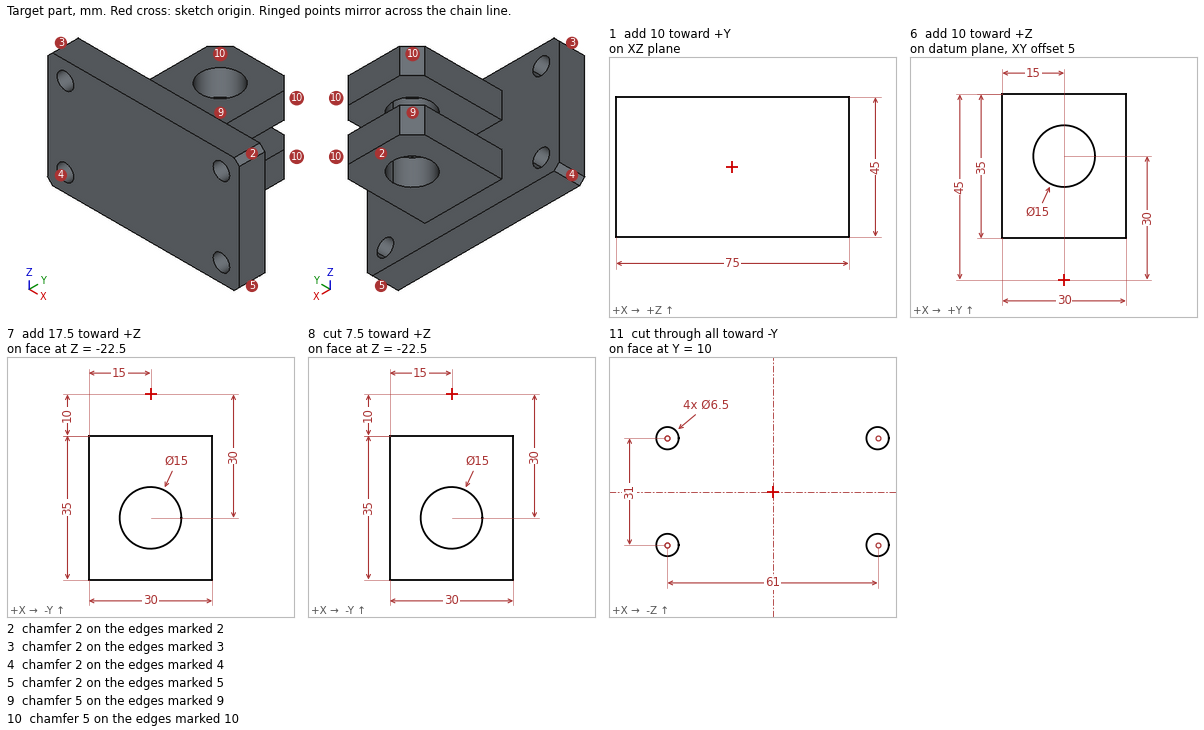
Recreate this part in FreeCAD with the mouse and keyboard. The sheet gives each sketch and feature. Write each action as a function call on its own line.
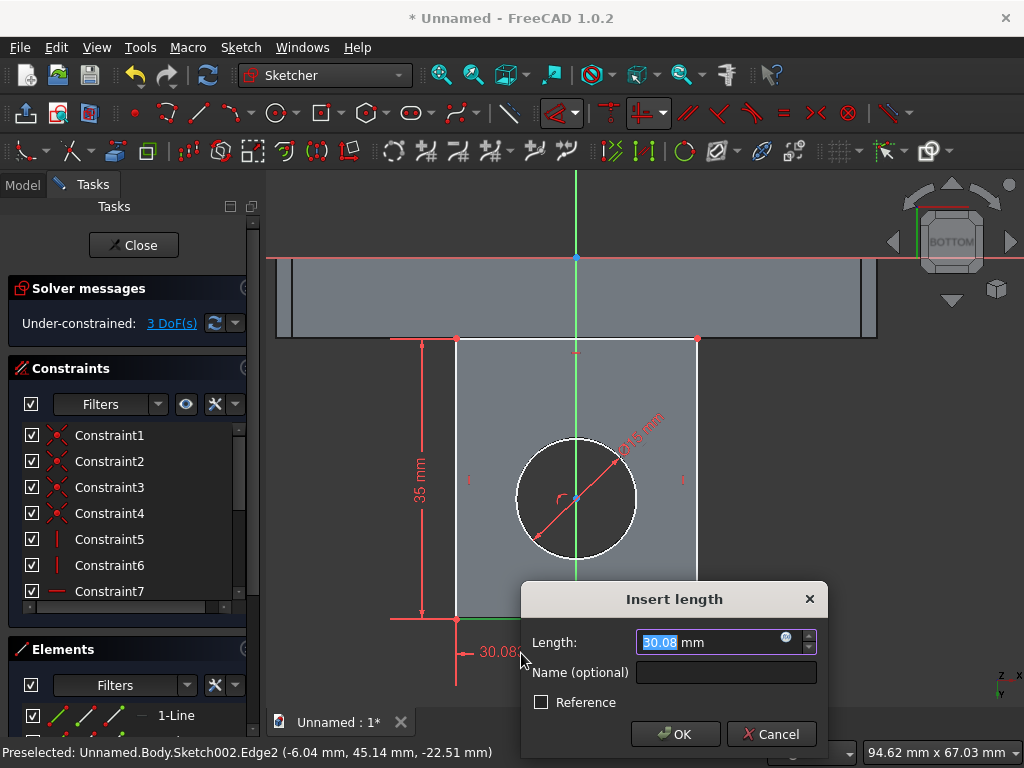
text(30)
key(Return)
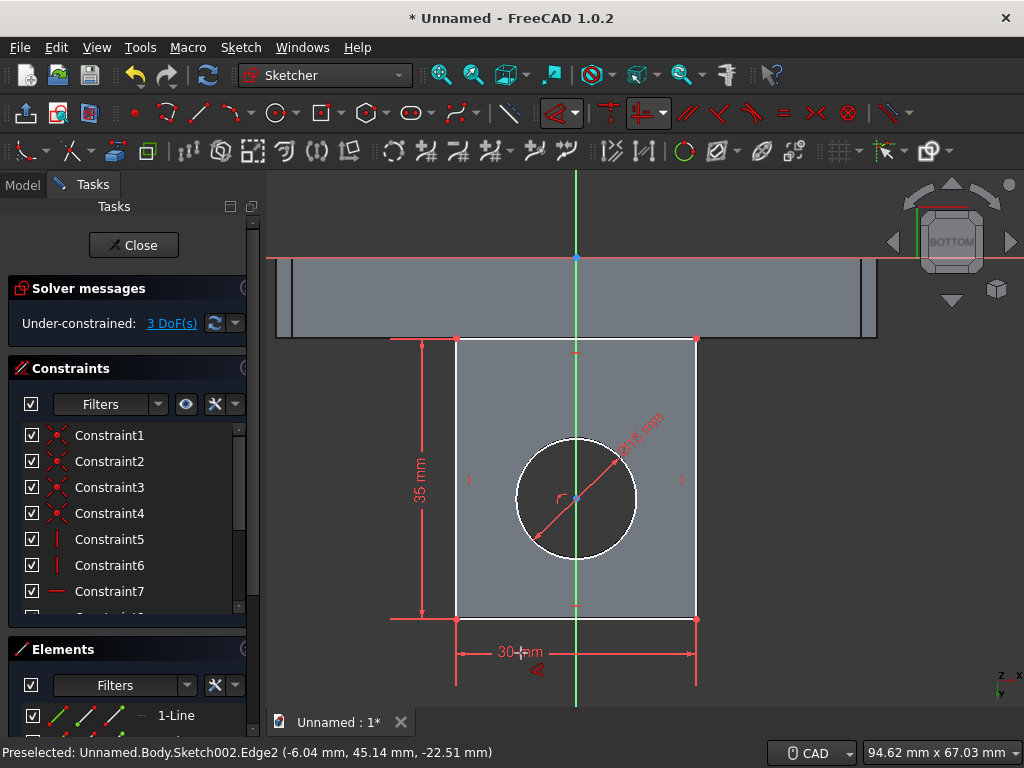
click(576, 499)
click(610, 378)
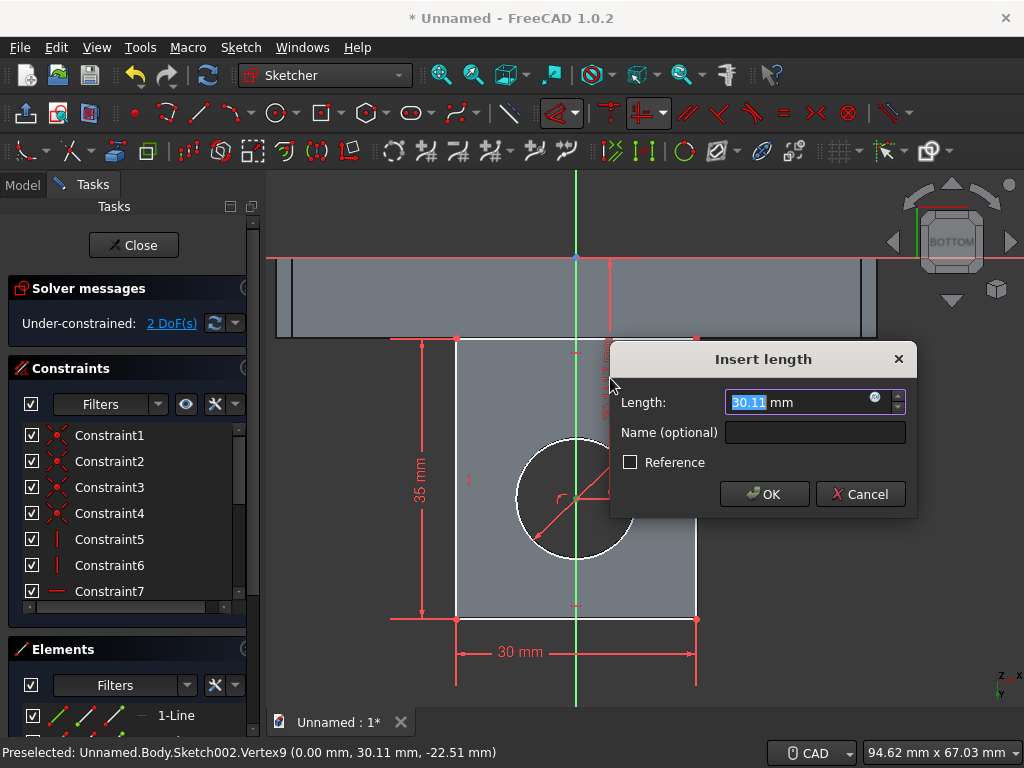
text(30)
key(Return)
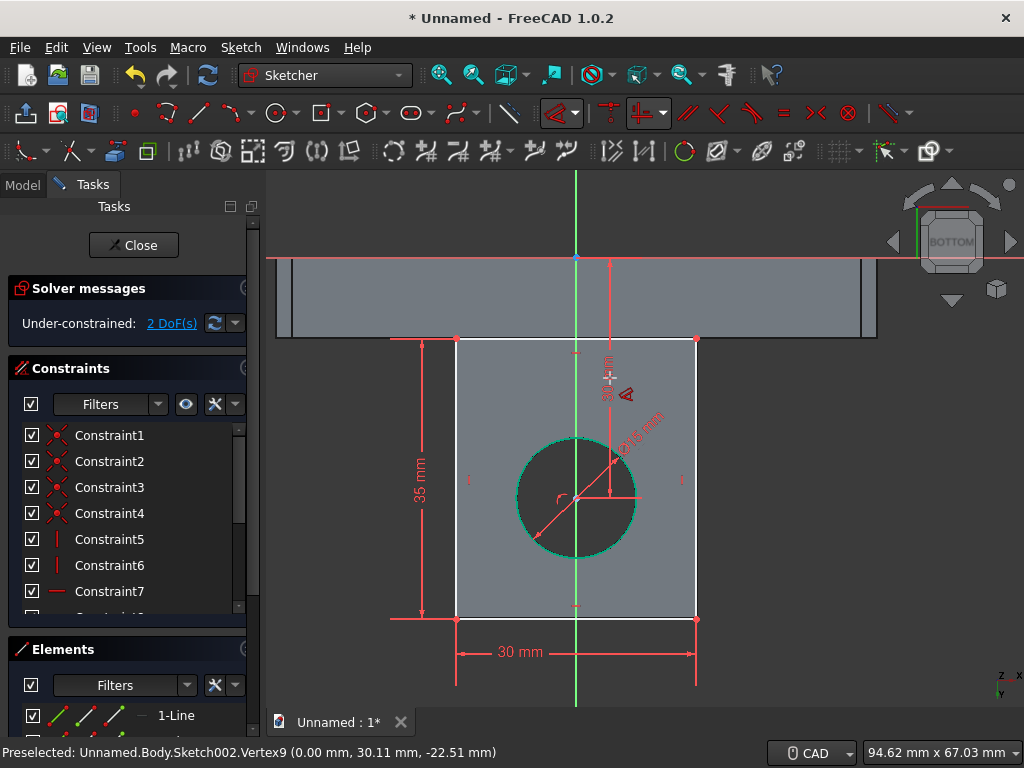
click(456, 339)
click(516, 224)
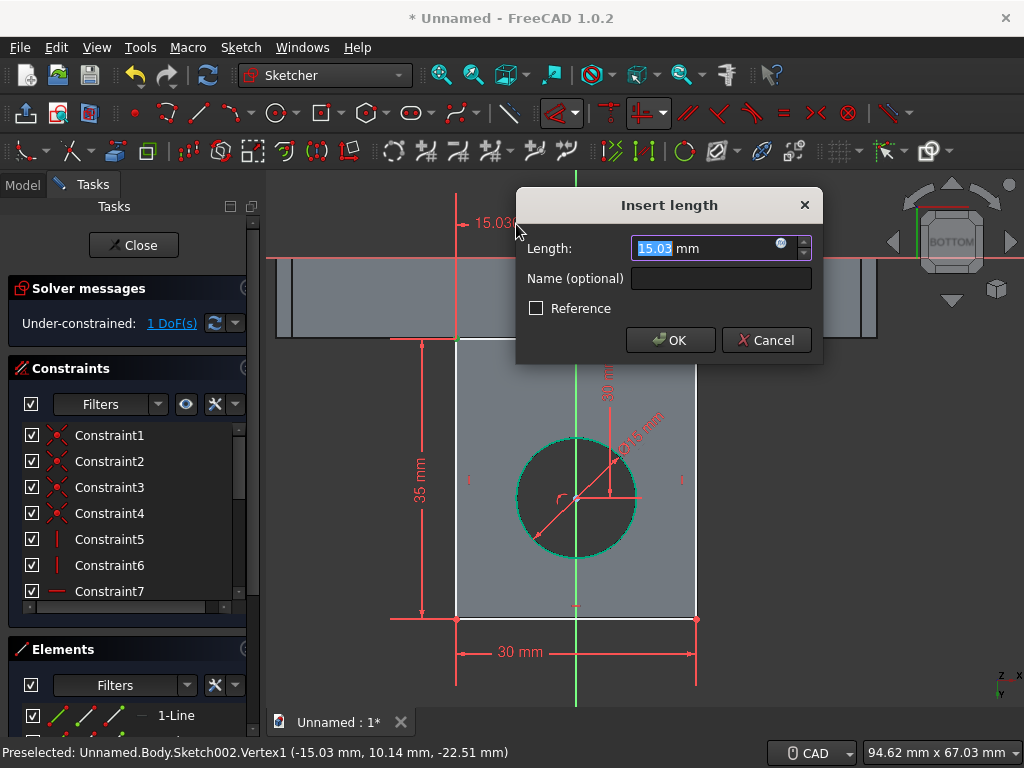
text(15)
key(Return)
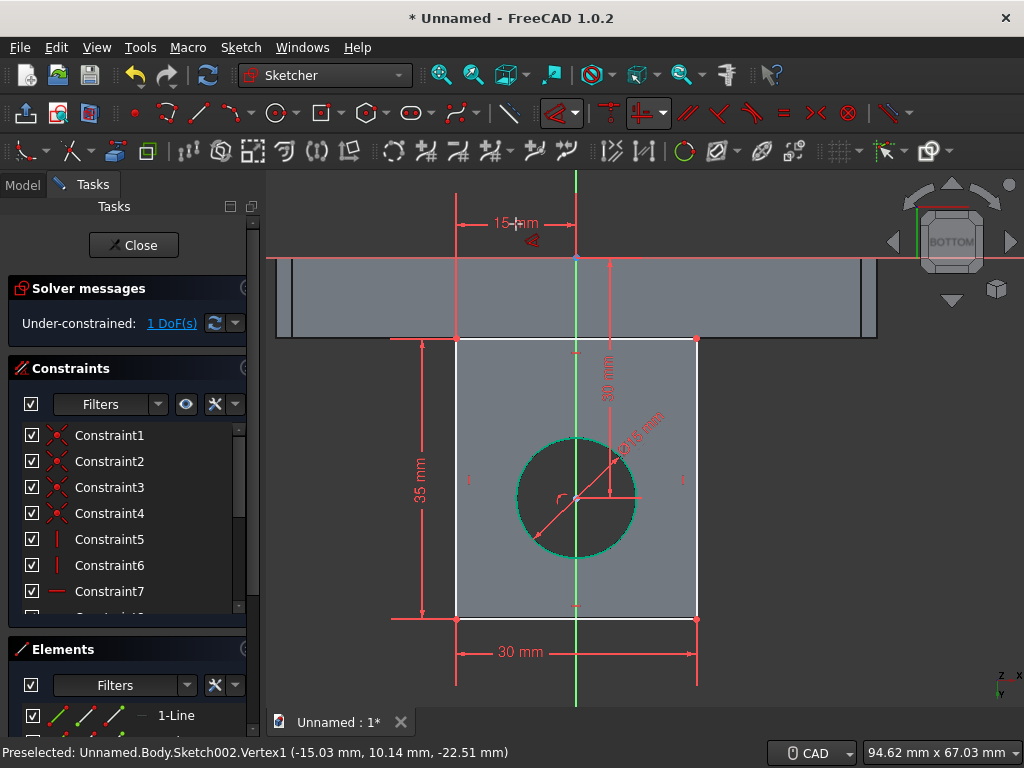
click(456, 339)
click(422, 298)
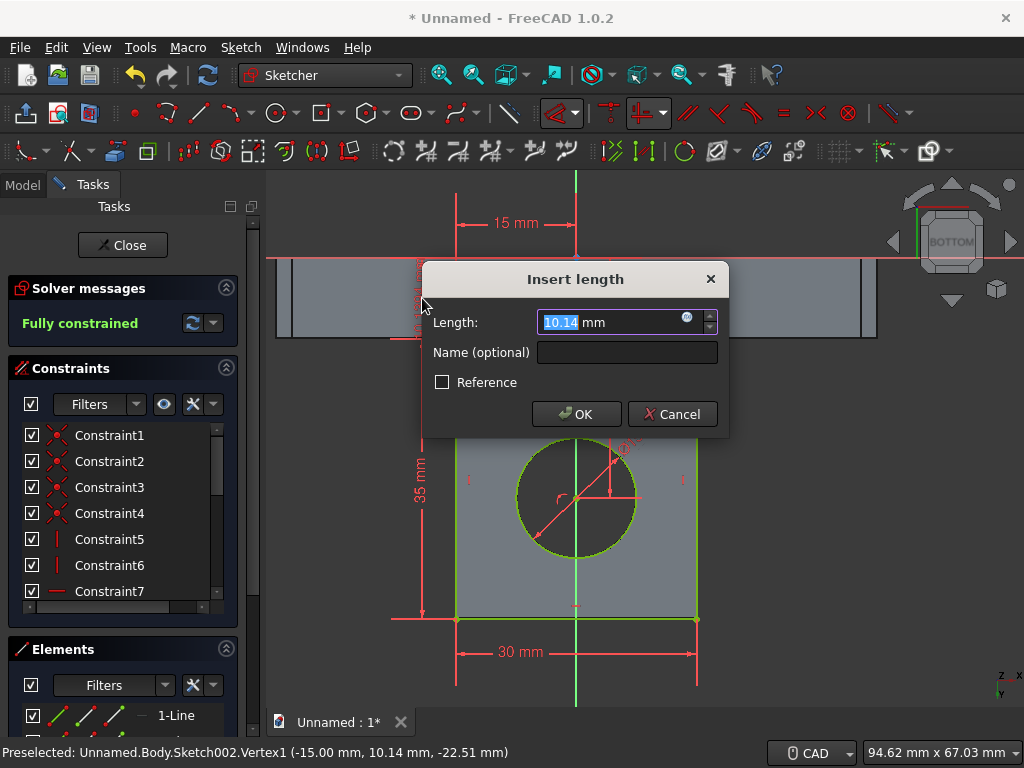
text(10)
key(Return)
key(Escape)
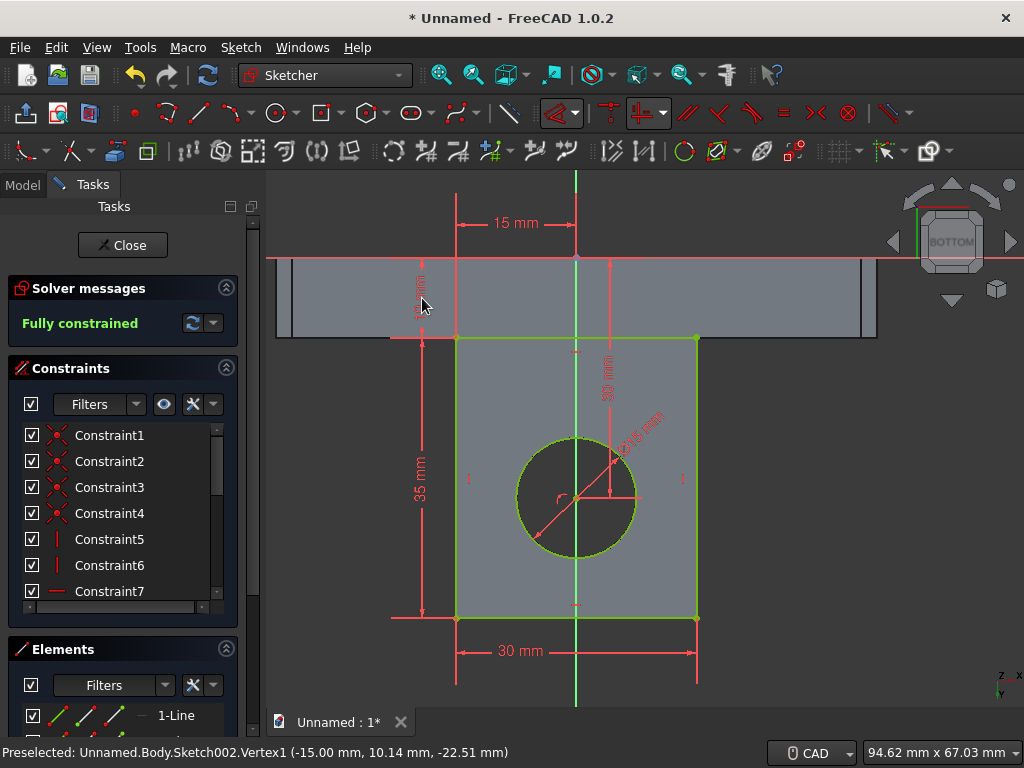
click(123, 245)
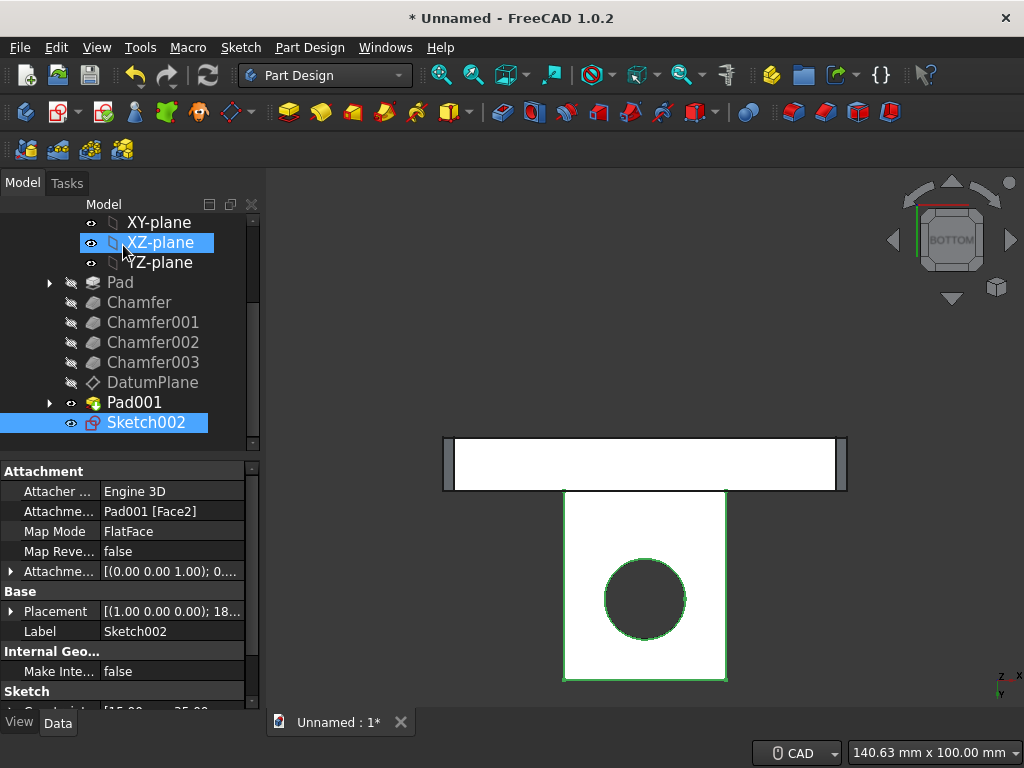
click(290, 112)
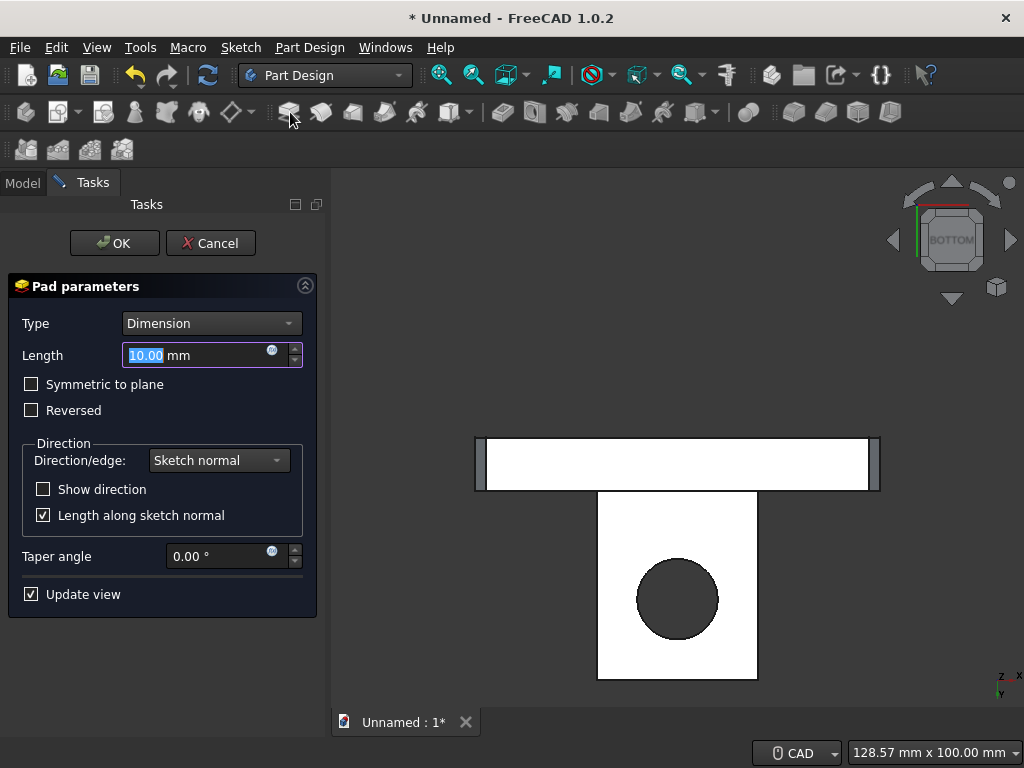
text(17.5)
key(Tab)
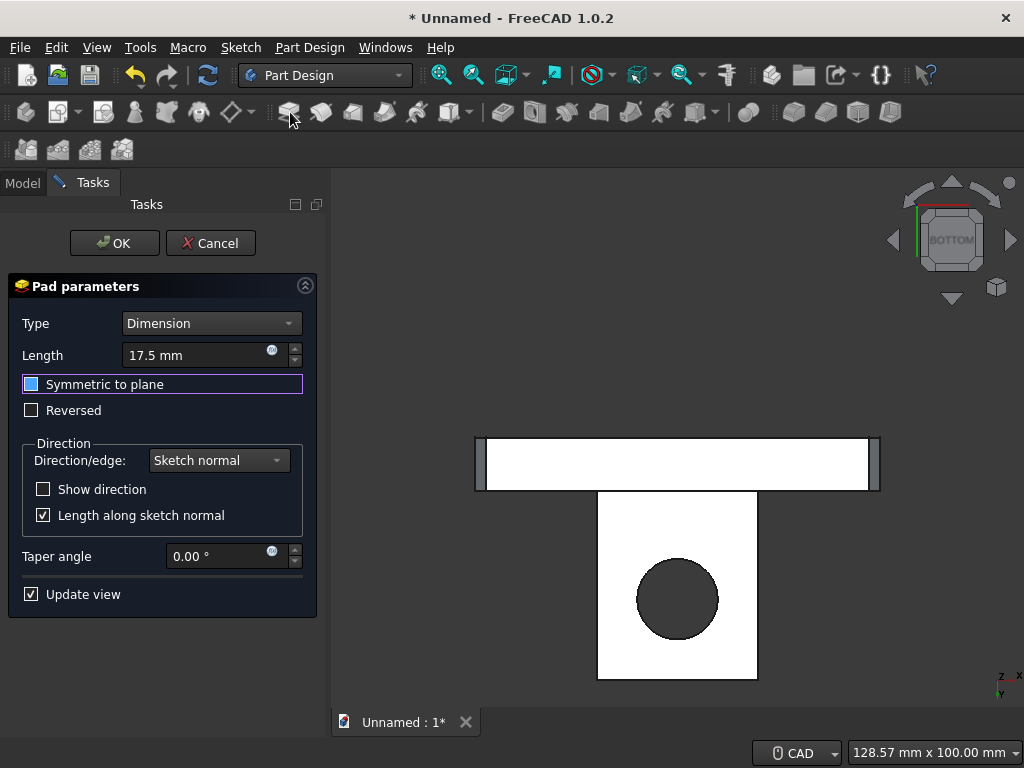
click(30, 410)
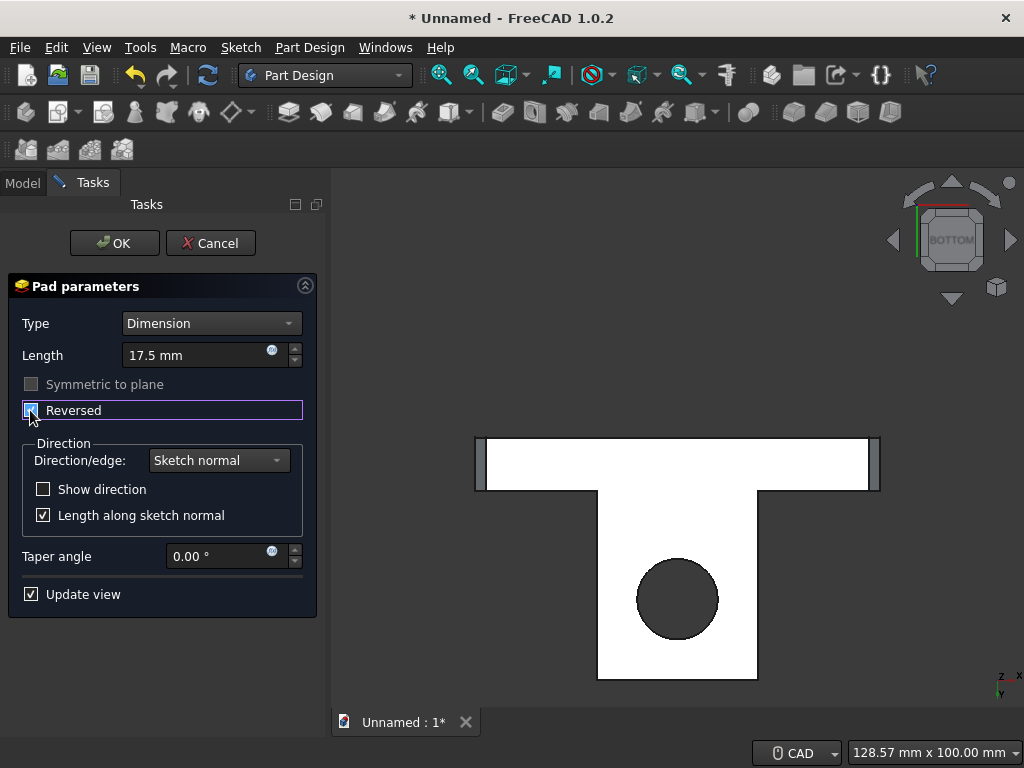
click(115, 243)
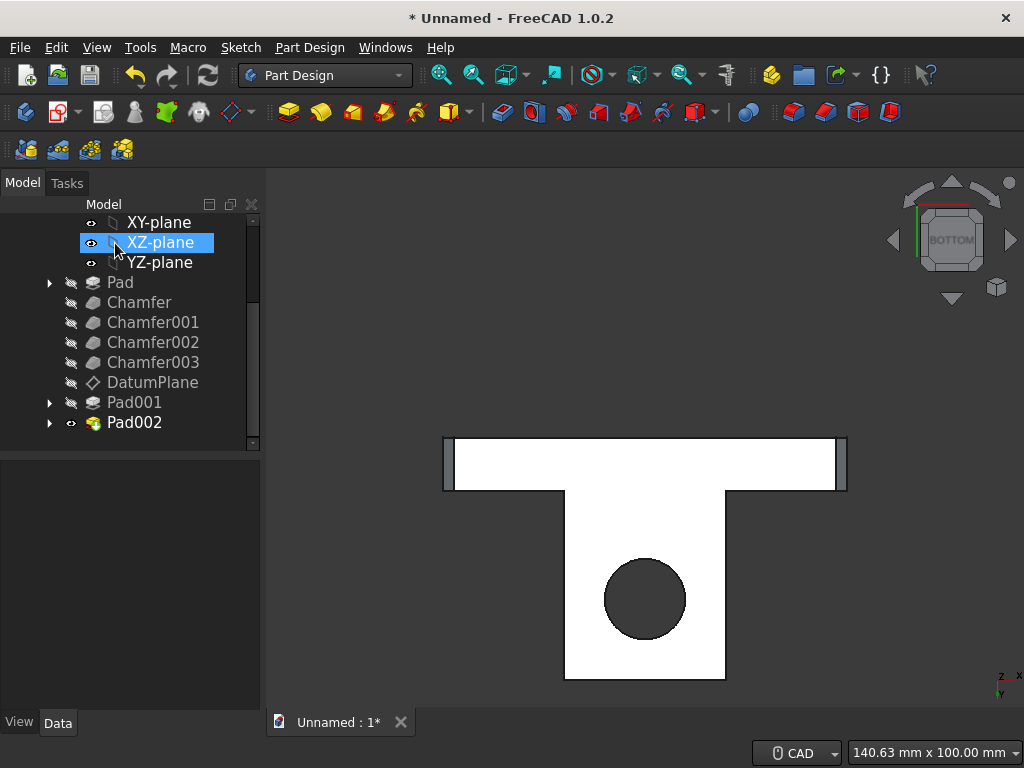
click(645, 488)